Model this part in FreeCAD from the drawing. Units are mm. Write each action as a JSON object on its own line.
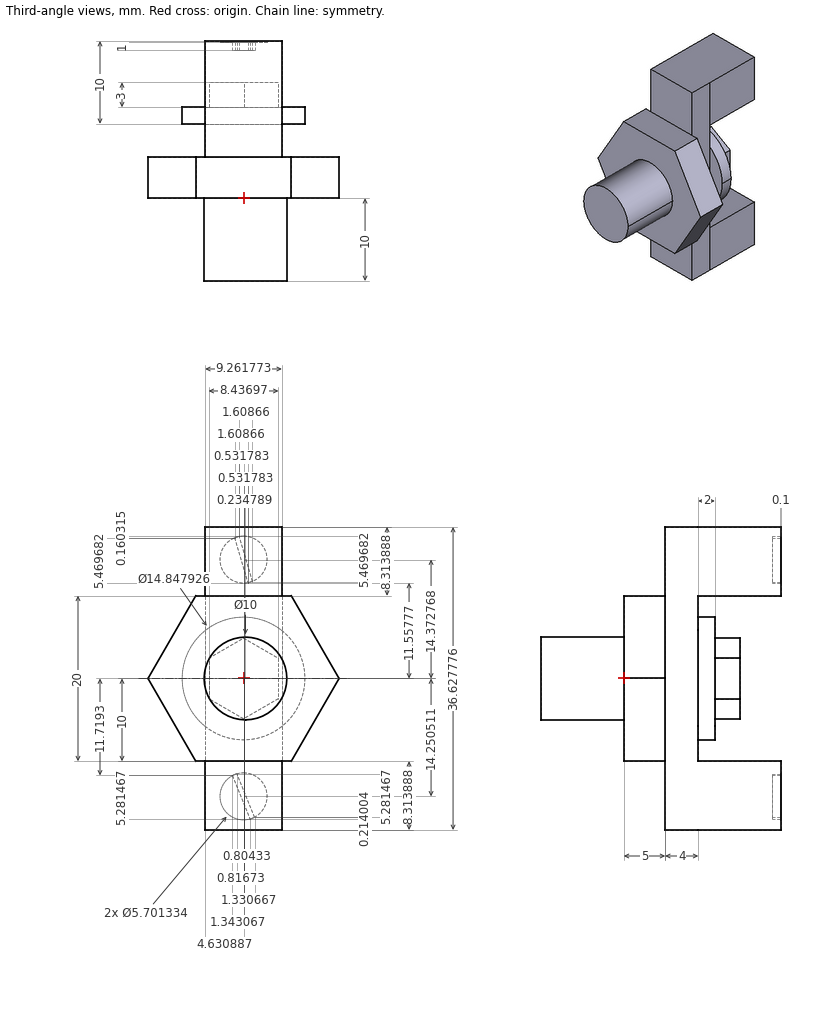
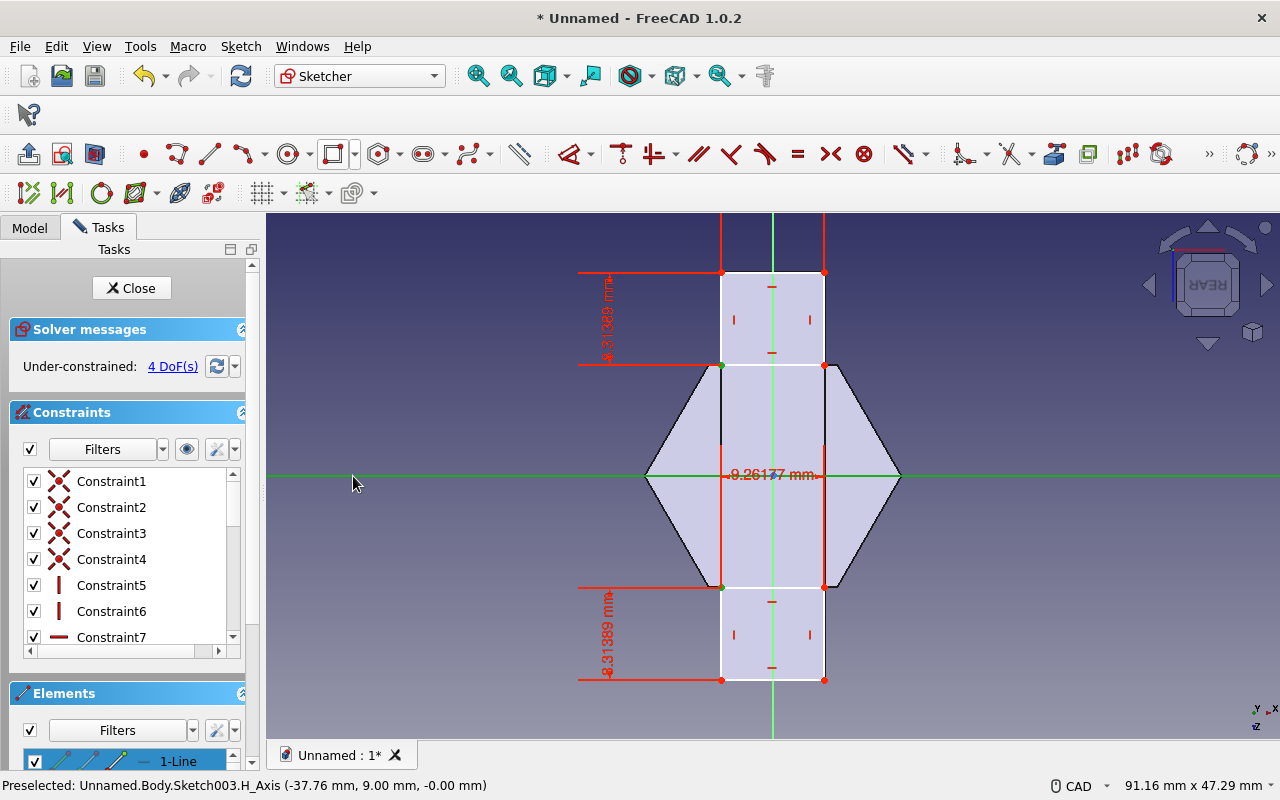
{"action": "left_click", "coordinate": [831, 154]}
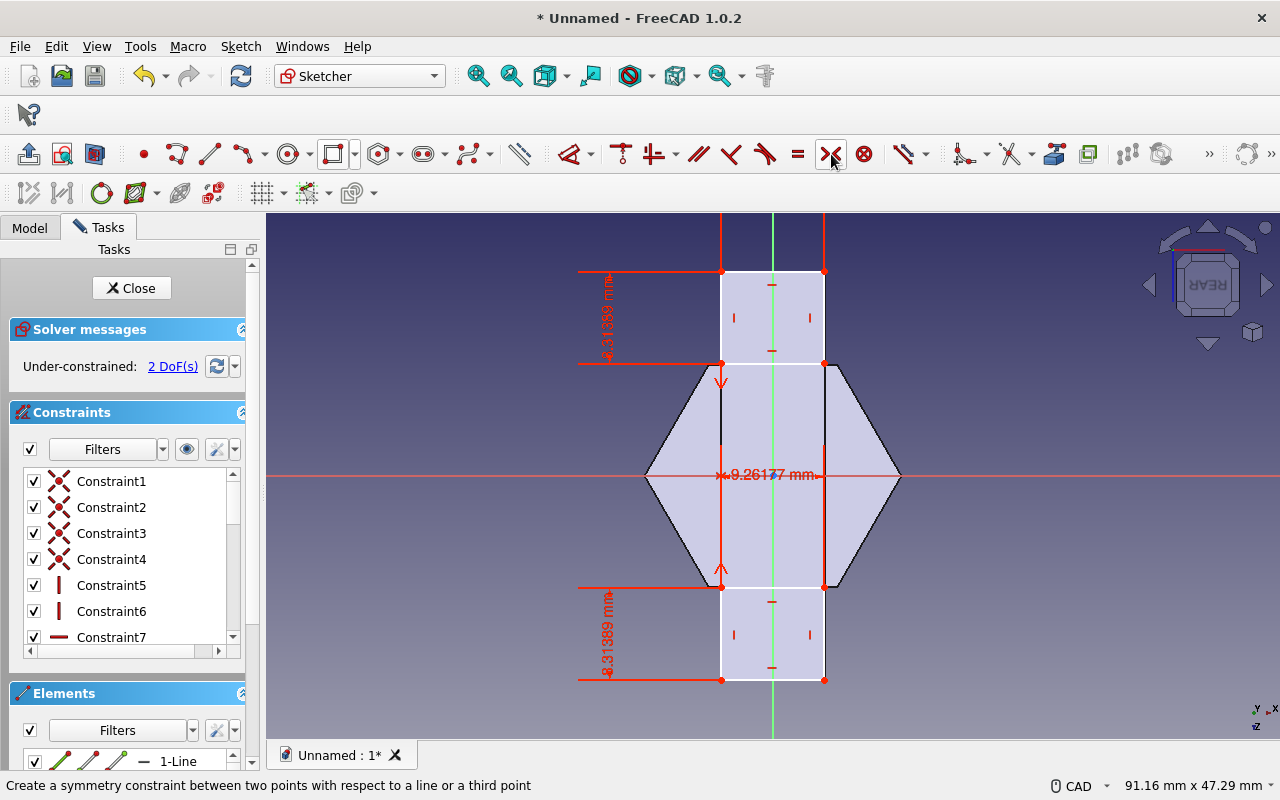
{"action": "left_click", "coordinate": [568, 154]}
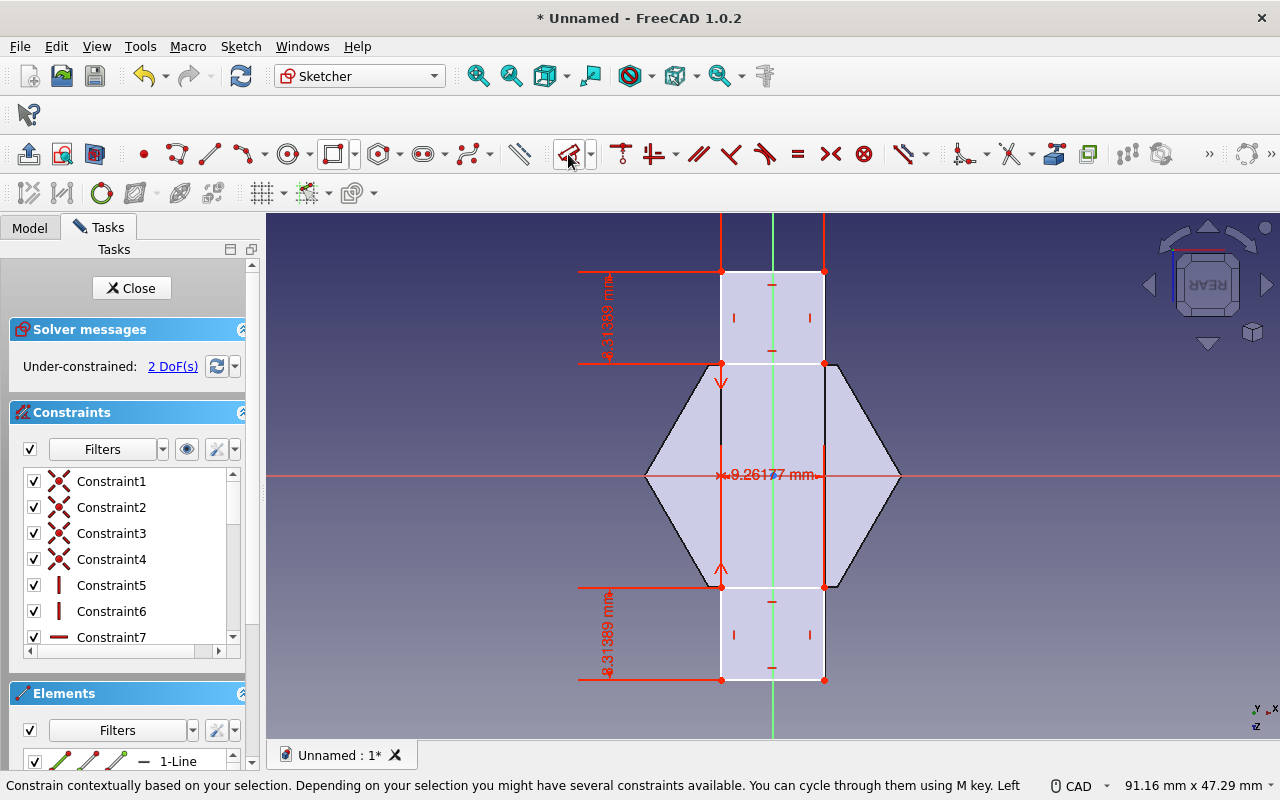
{"action": "left_click", "coordinate": [721, 364]}
{"action": "left_click", "coordinate": [687, 420]}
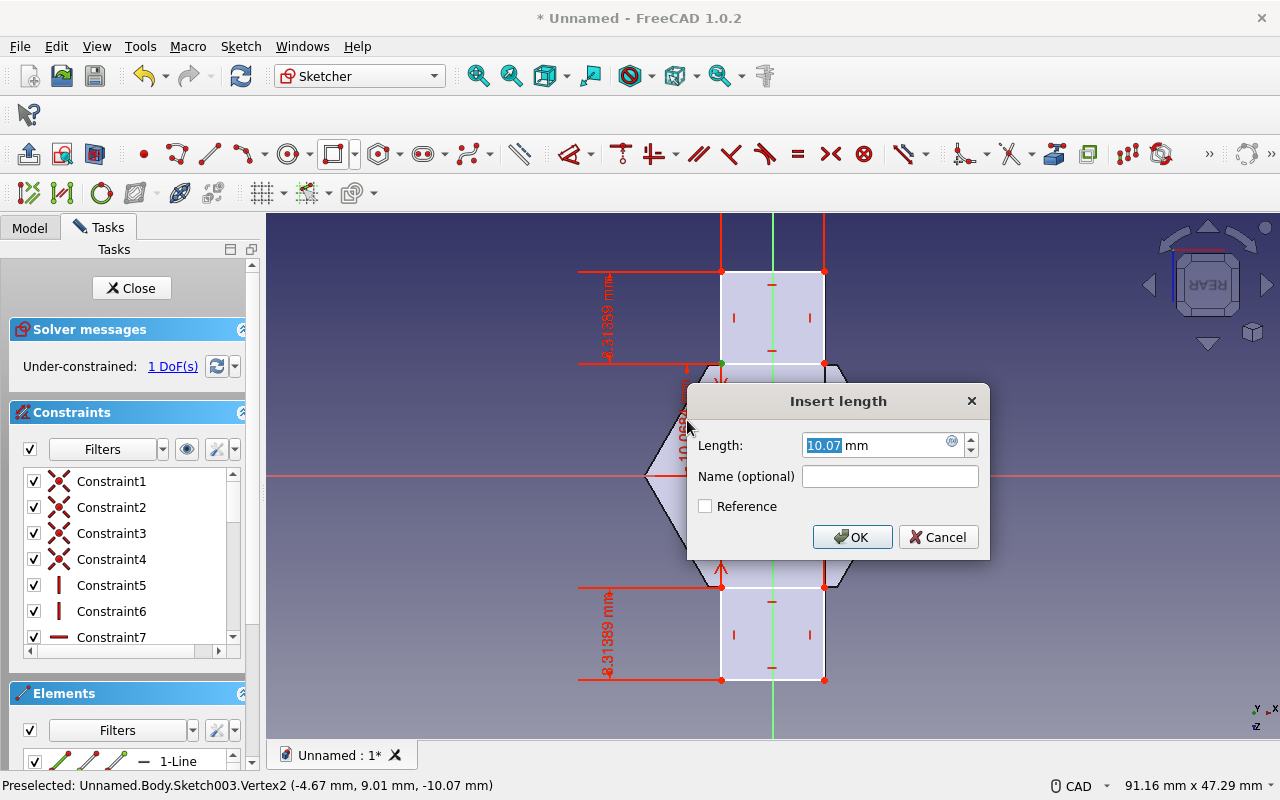
{"action": "type", "text": "10"}
{"action": "key", "text": "Return"}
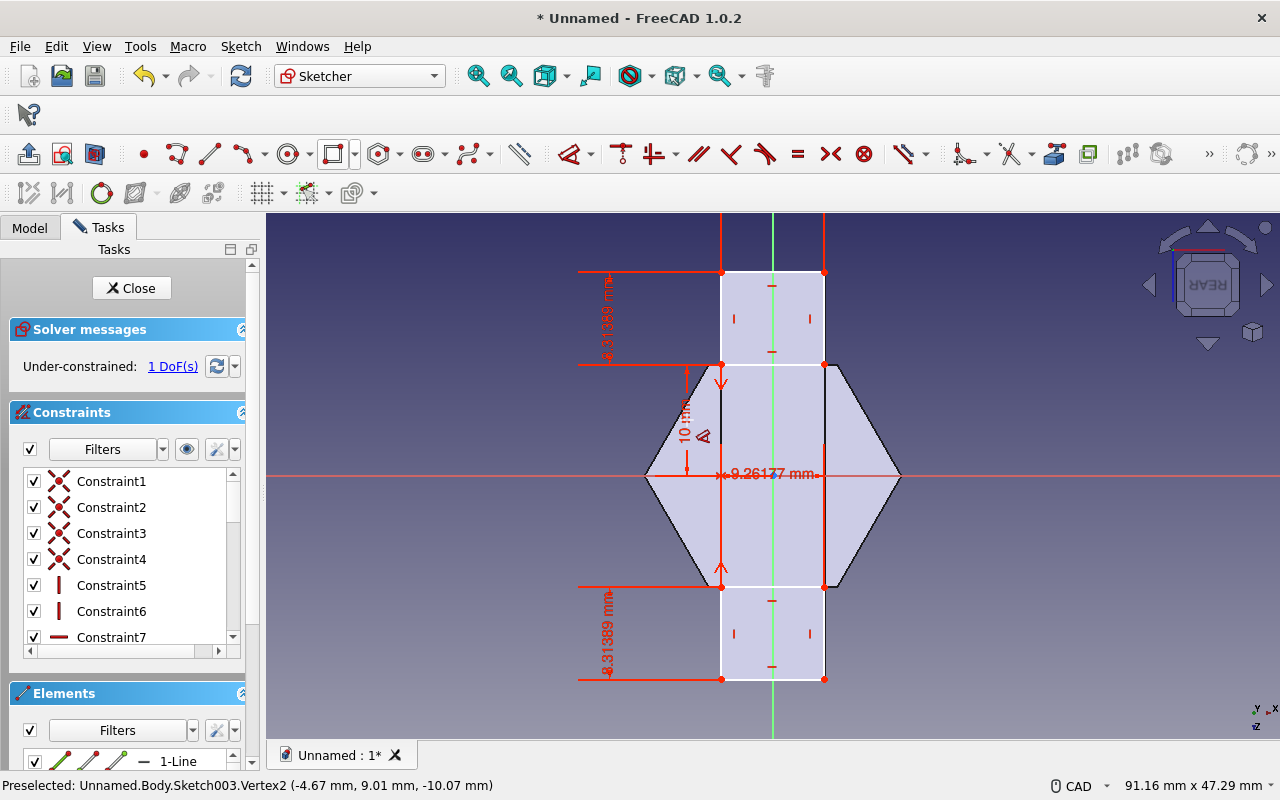
{"action": "left_click", "coordinate": [721, 272]}
{"action": "left_click", "coordinate": [747, 510]}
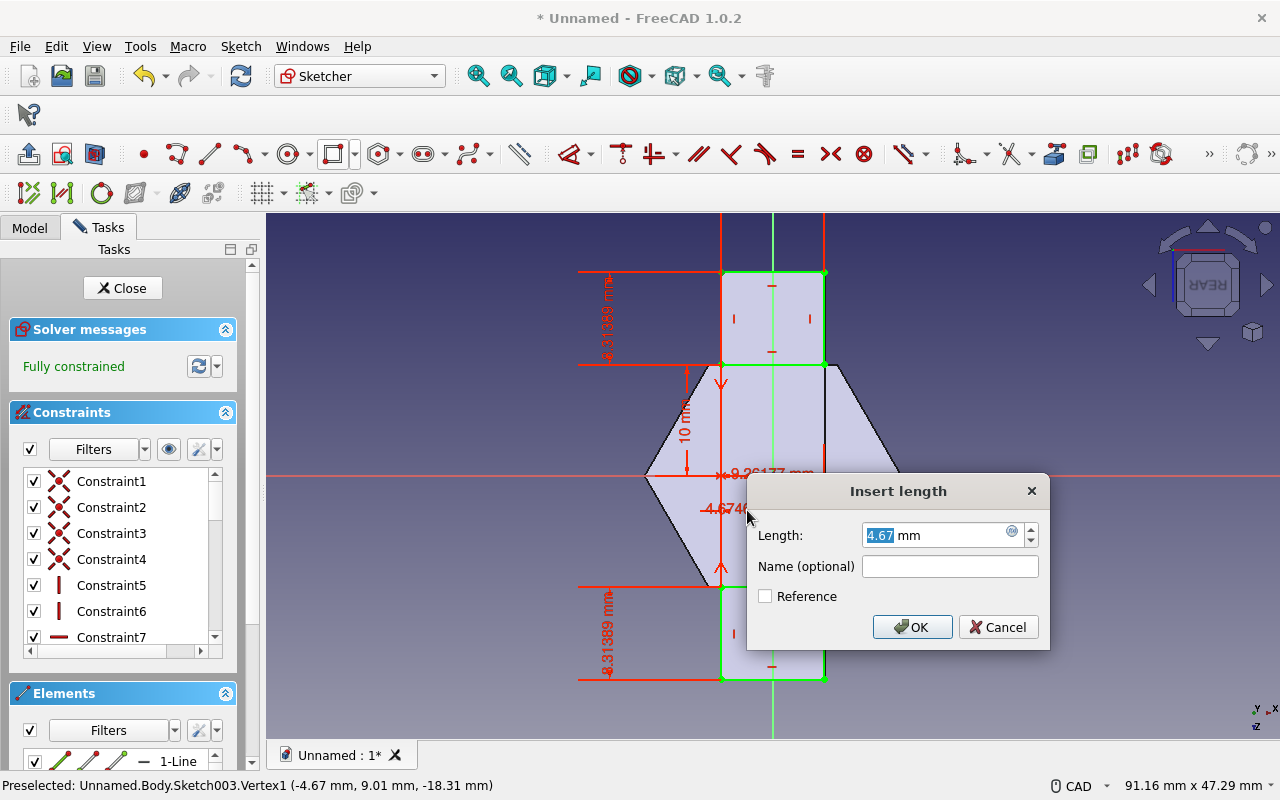
{"action": "type", "text": "4.630887"}
{"action": "key", "text": "Return"}
{"action": "key", "text": "Escape"}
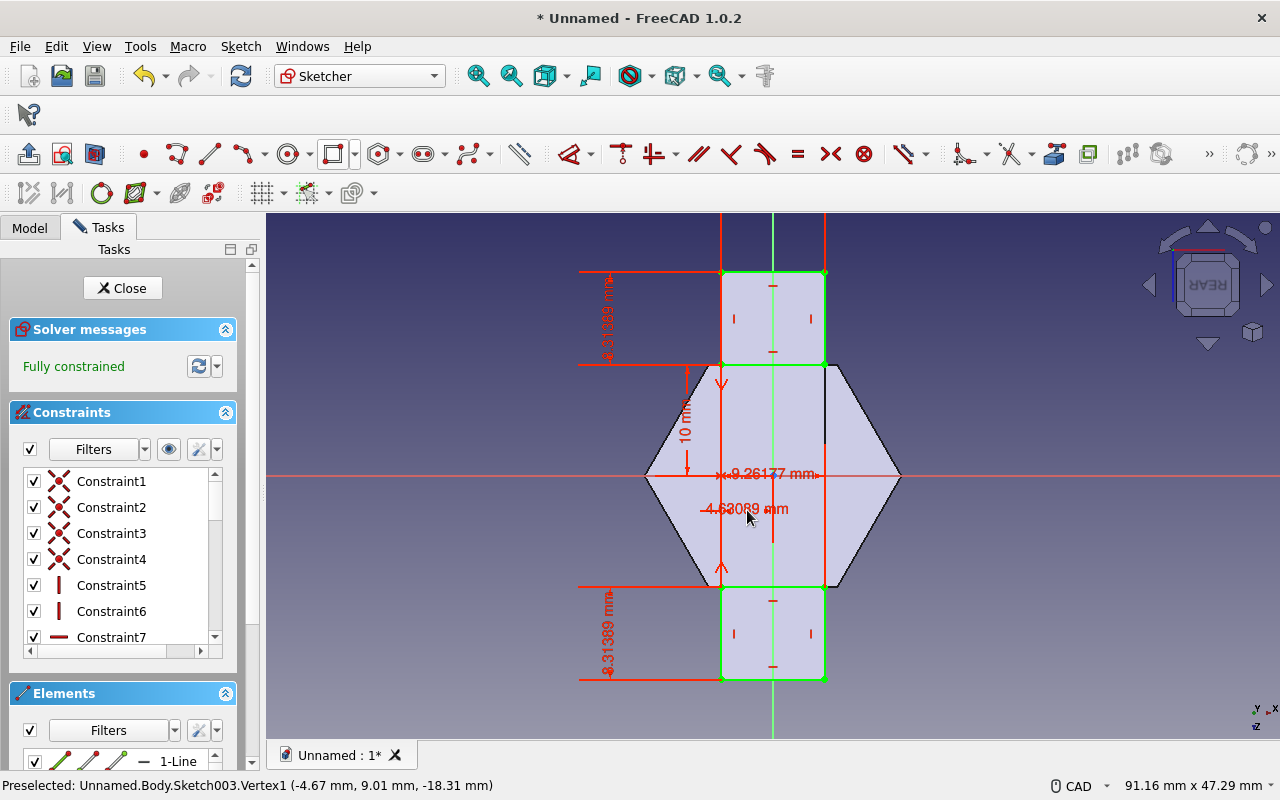
{"action": "left_click", "coordinate": [123, 288]}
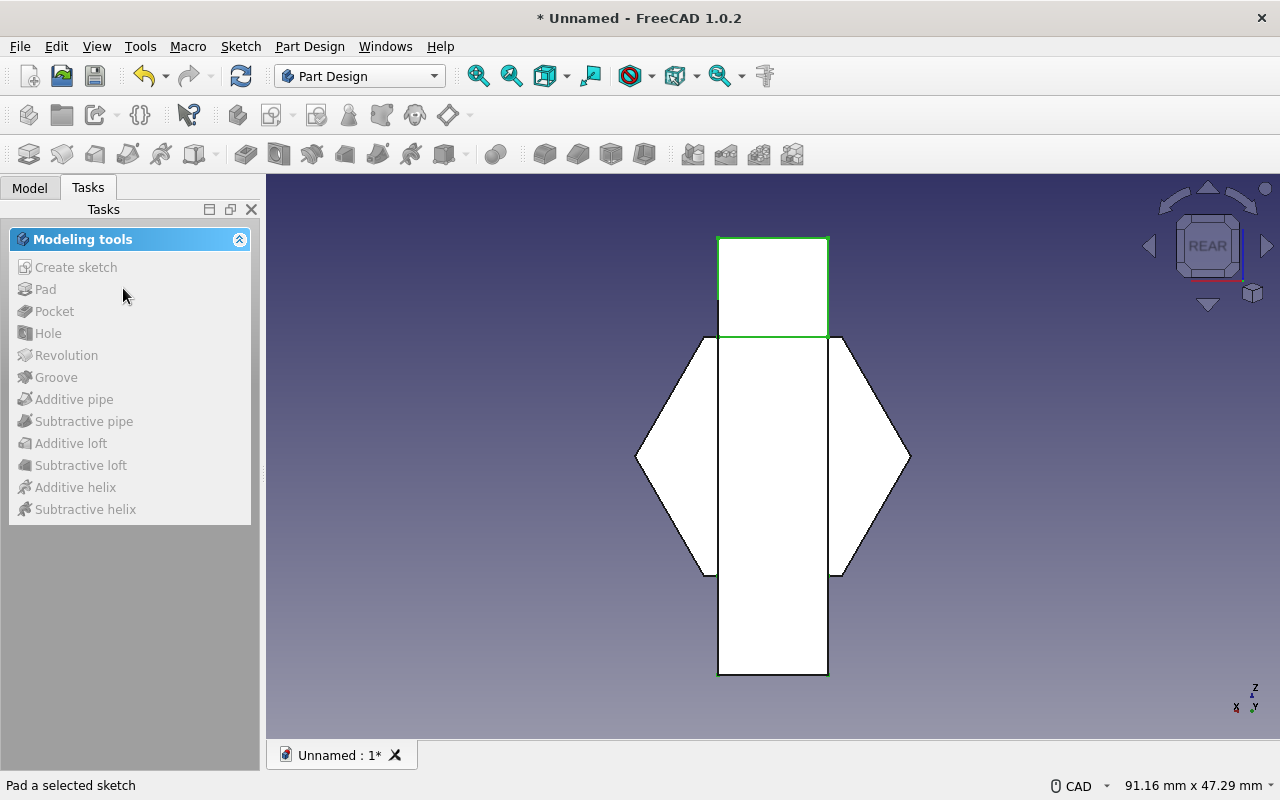
{"action": "left_click", "coordinate": [29, 154]}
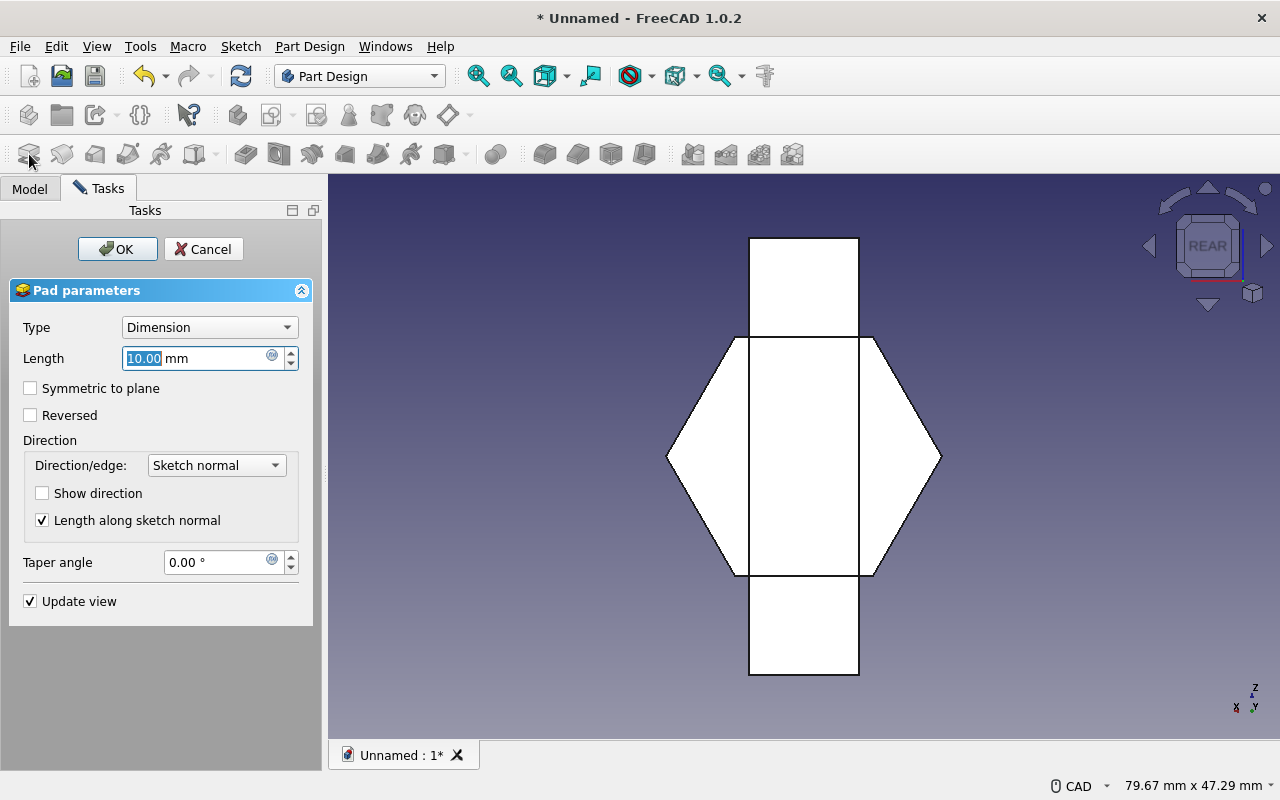
{"action": "type", "text": "10"}
{"action": "key", "text": "Tab"}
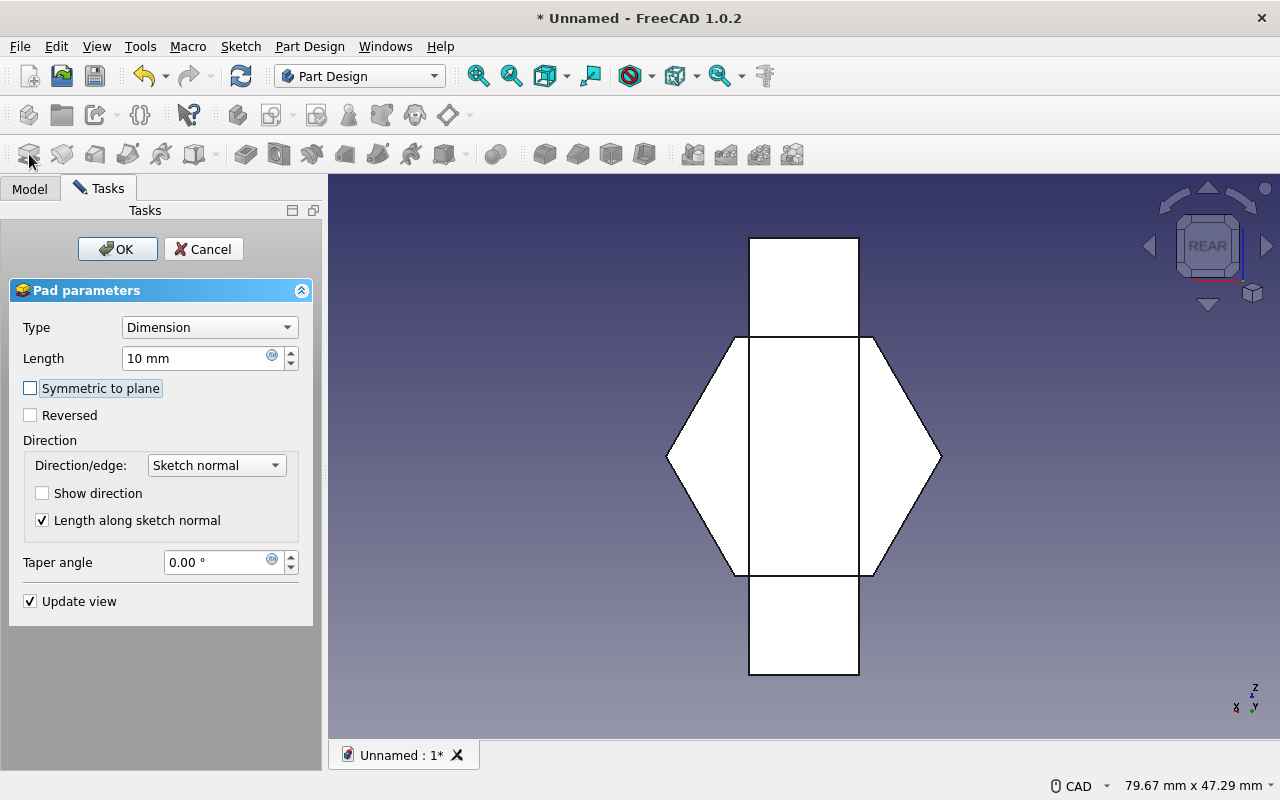
{"action": "left_click", "coordinate": [118, 249]}